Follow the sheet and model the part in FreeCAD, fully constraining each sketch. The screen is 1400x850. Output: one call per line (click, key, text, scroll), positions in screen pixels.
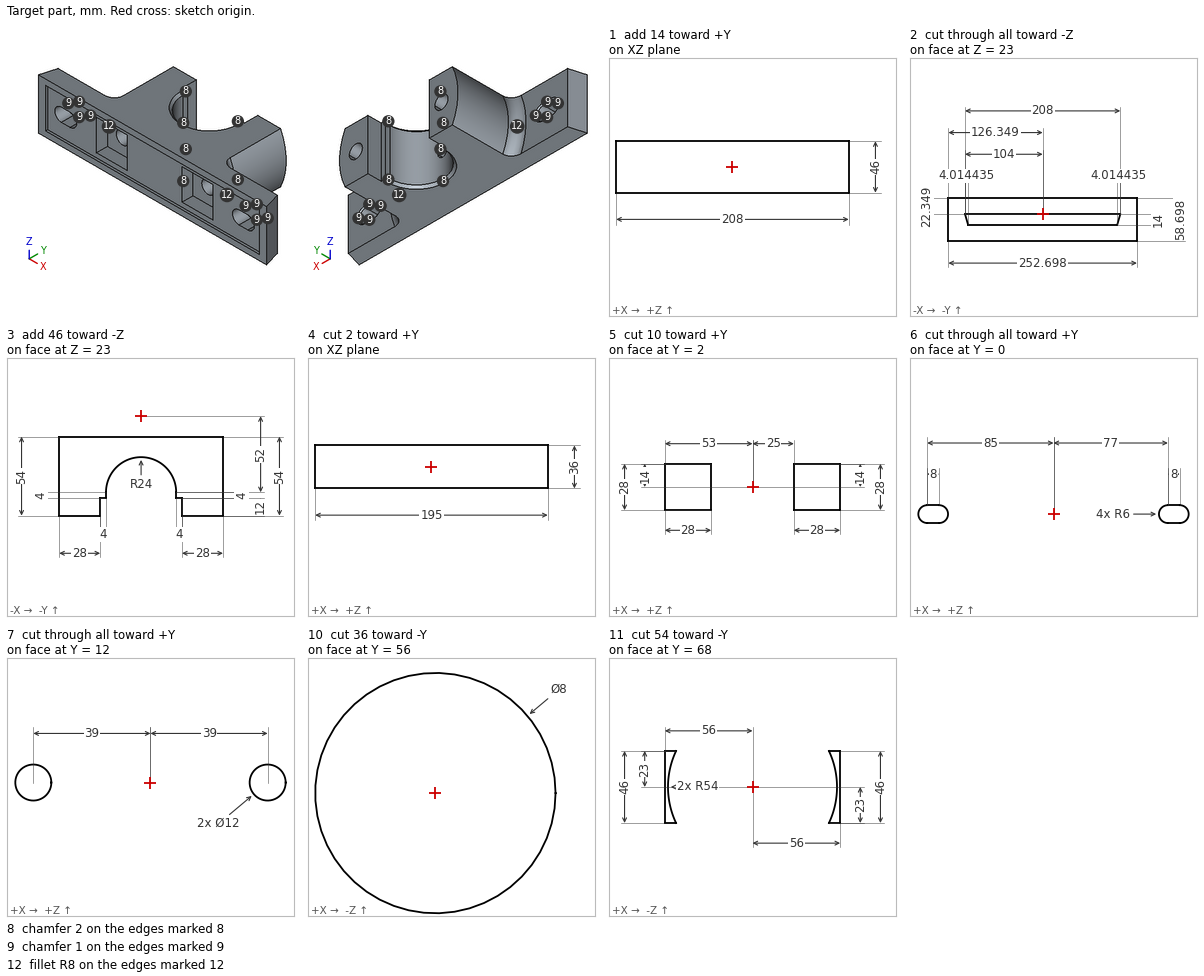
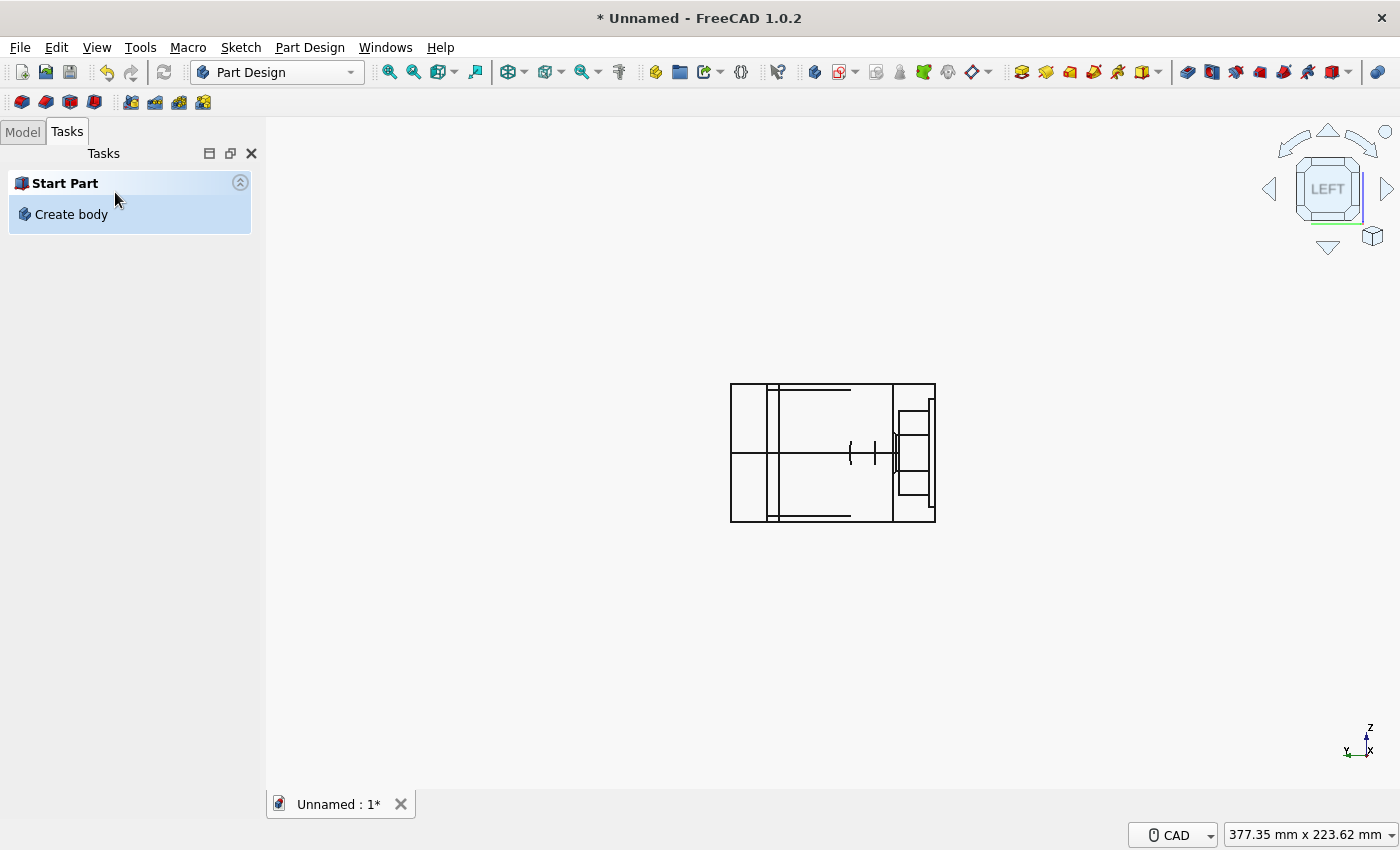
key(0)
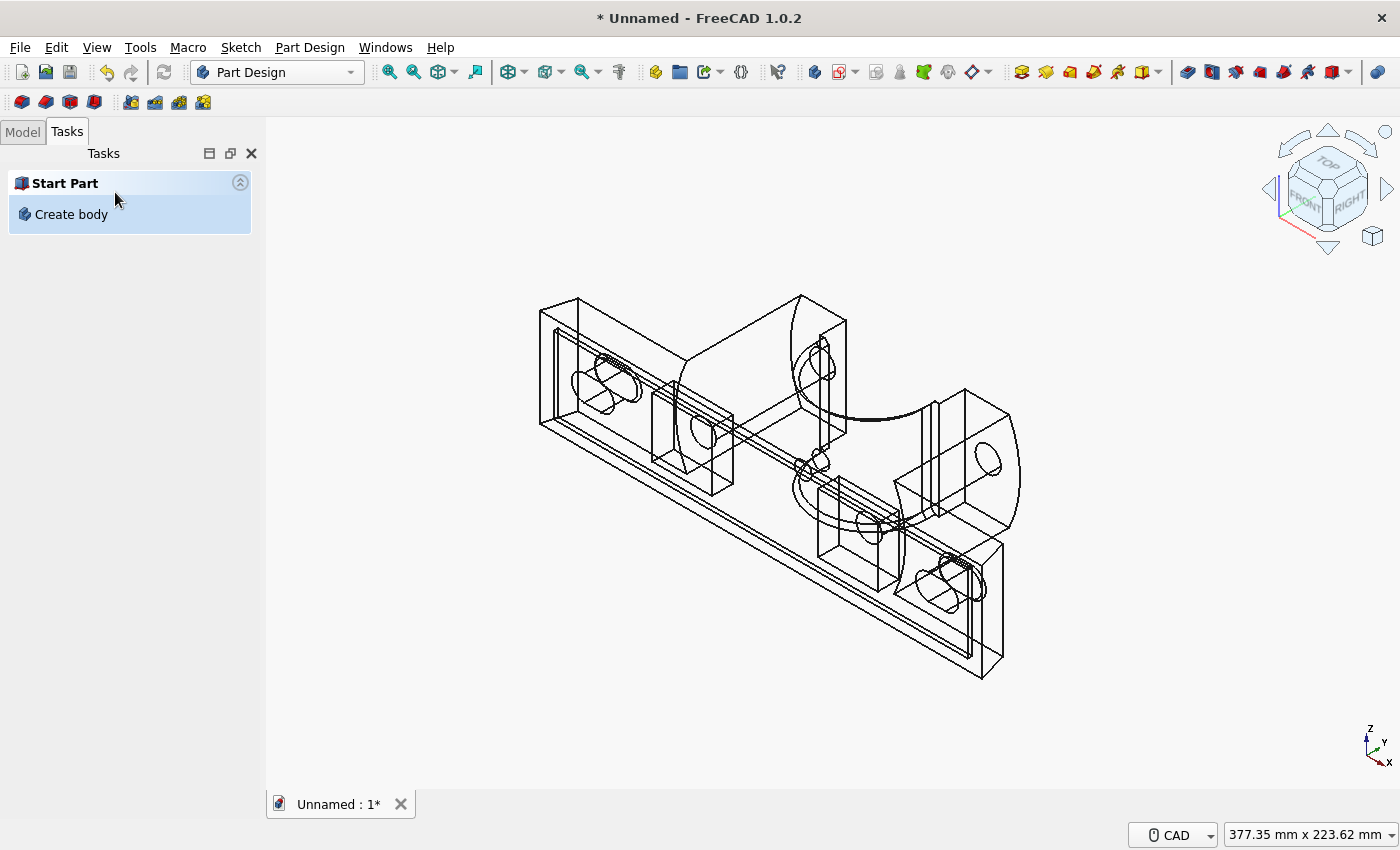
click(682, 370)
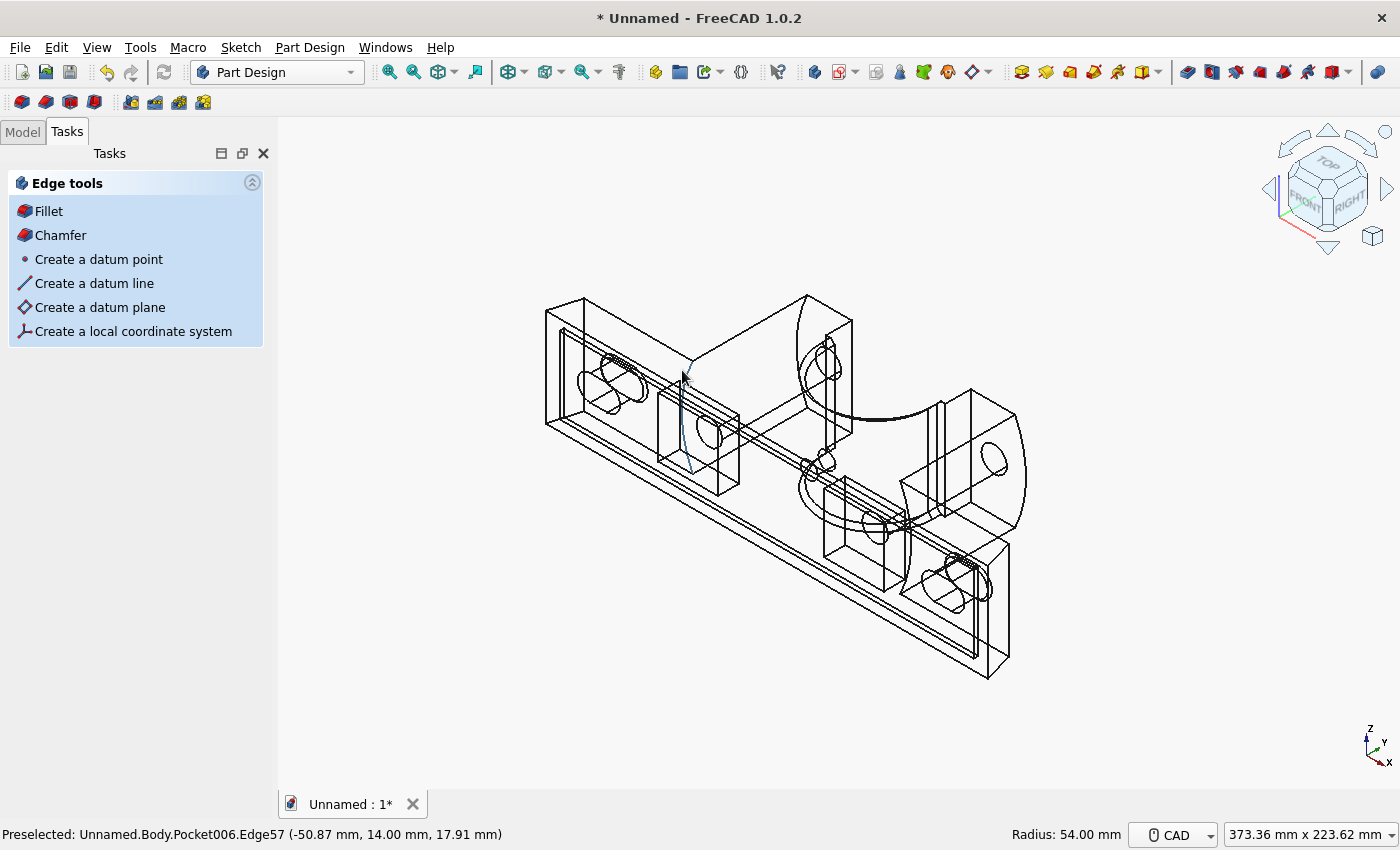
click(911, 543, ctrl)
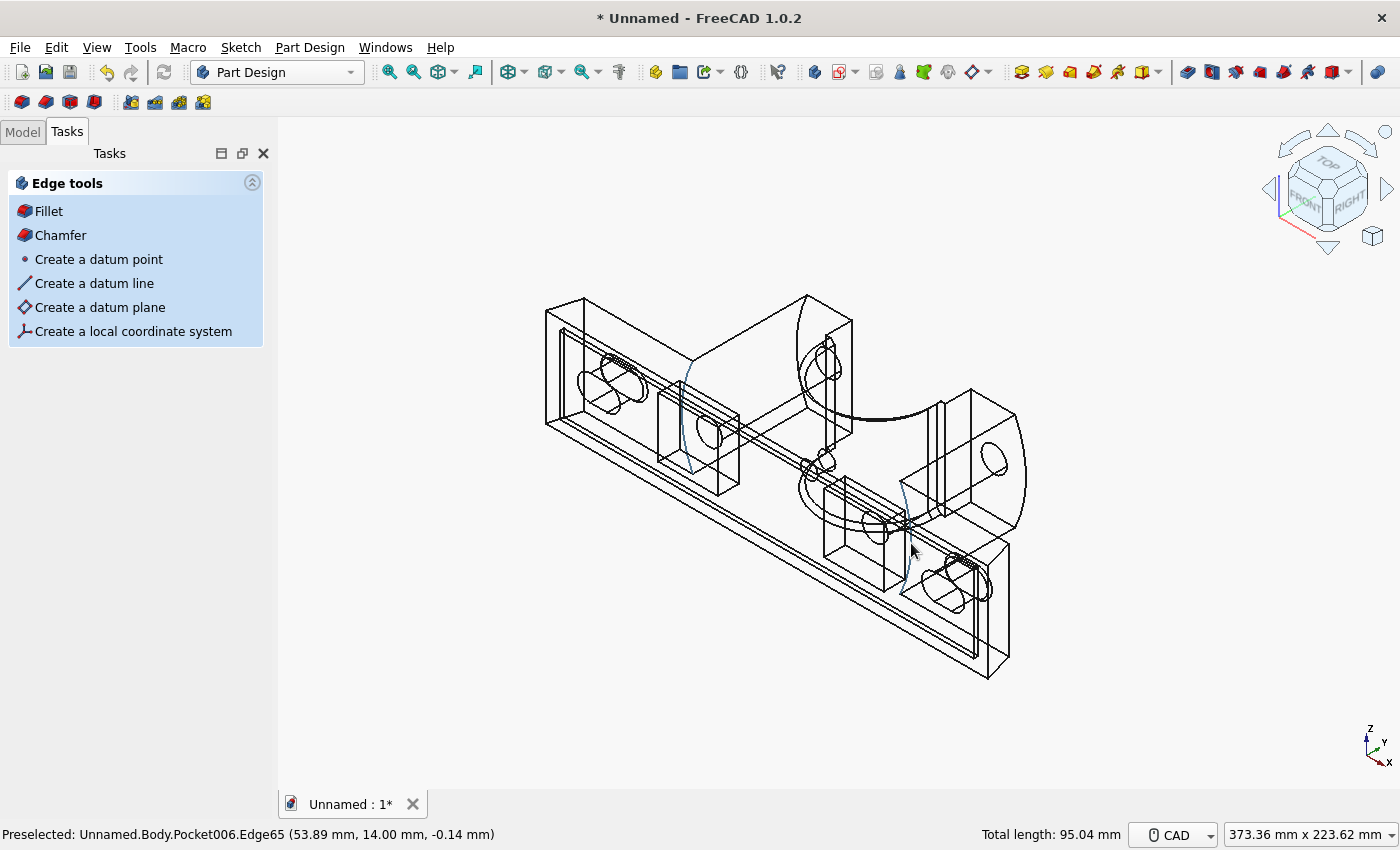
key(v)
key(1)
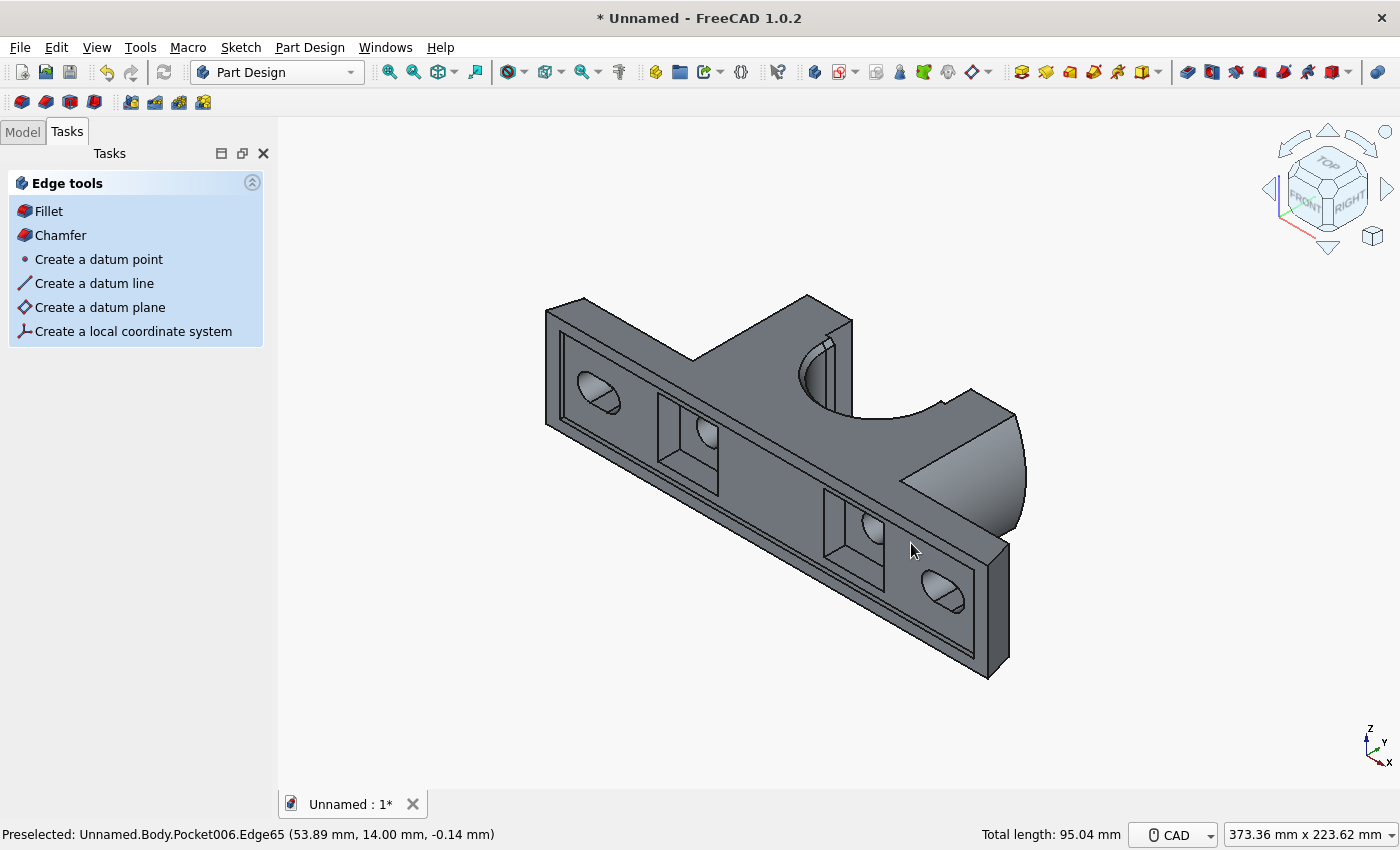
click(22, 102)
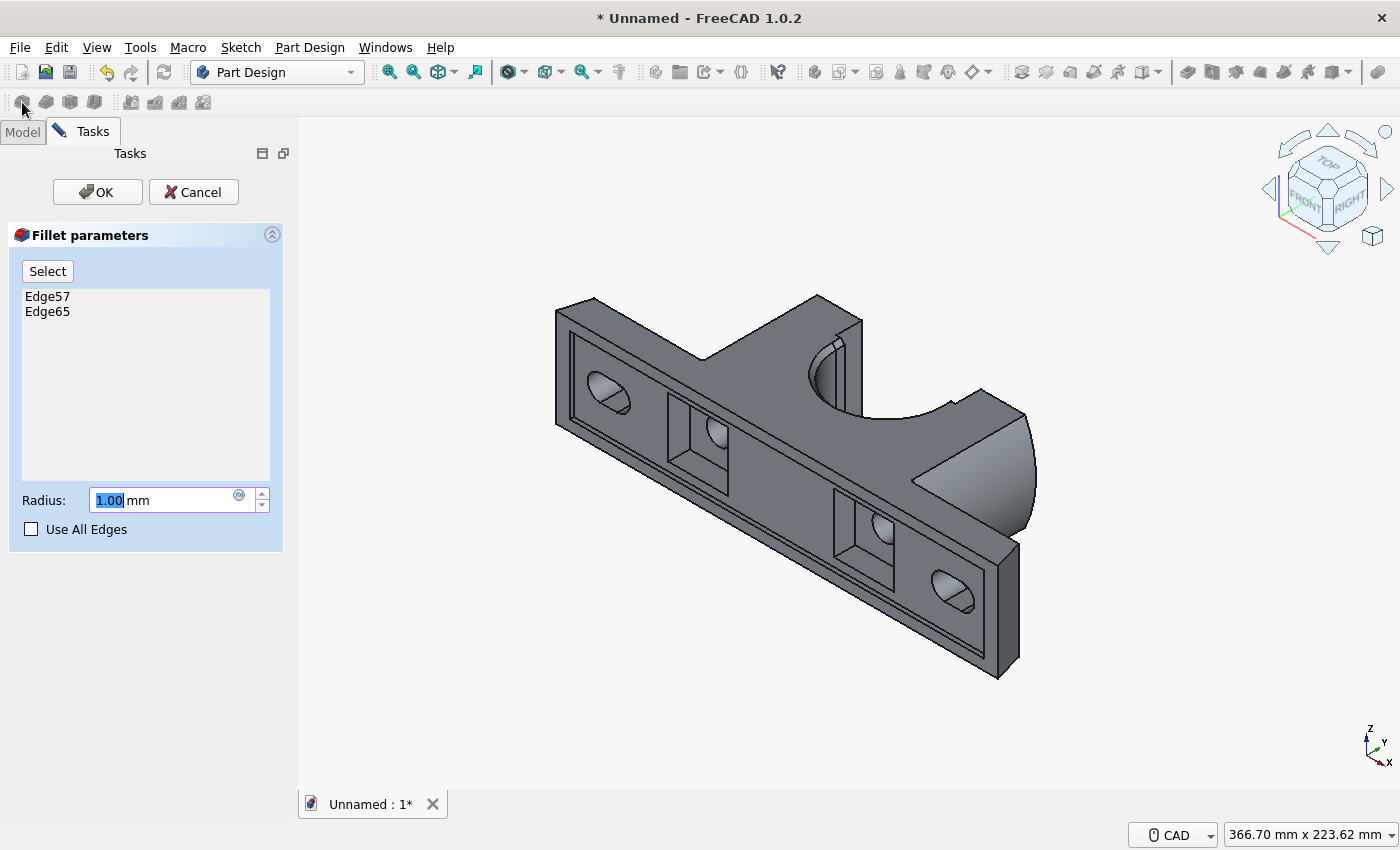
text(8)
key(Tab)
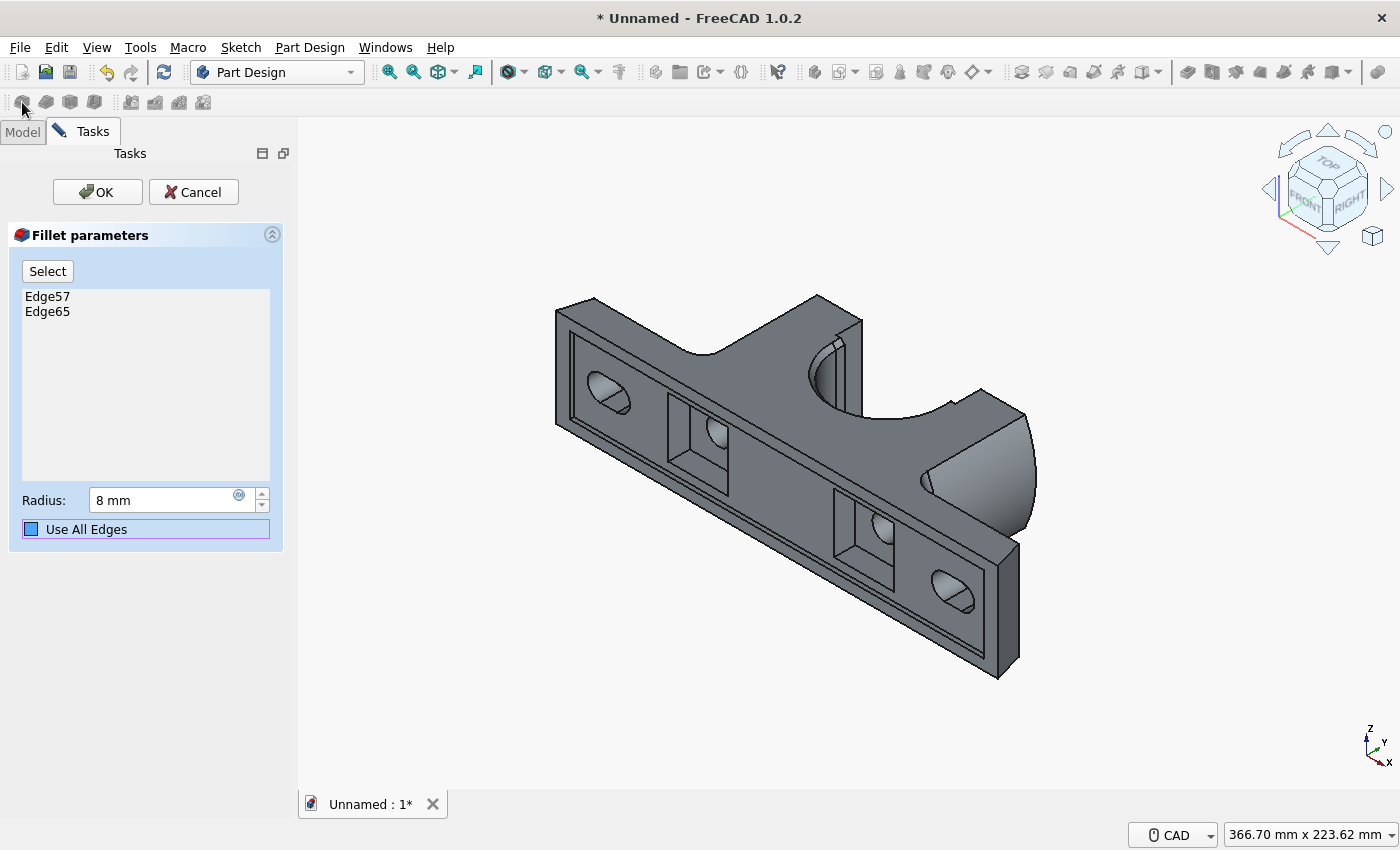
click(98, 192)